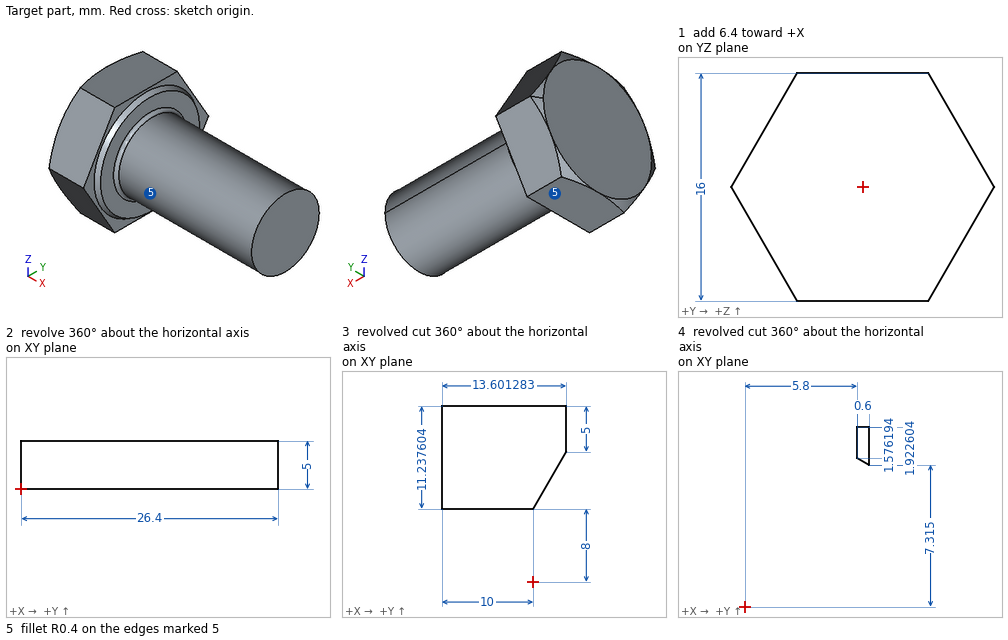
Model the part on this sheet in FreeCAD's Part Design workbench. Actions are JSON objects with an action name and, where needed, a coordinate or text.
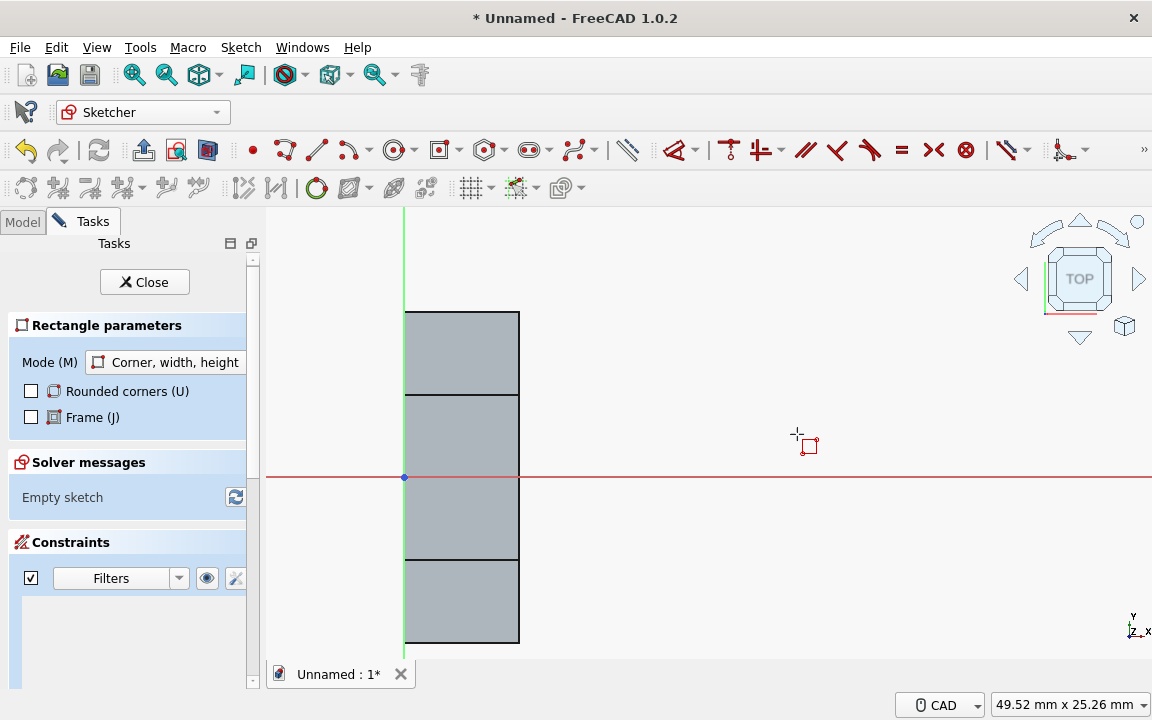
{"action": "left_click", "coordinate": [404, 477]}
{"action": "left_click", "coordinate": [876, 388]}
{"action": "key", "text": "Escape"}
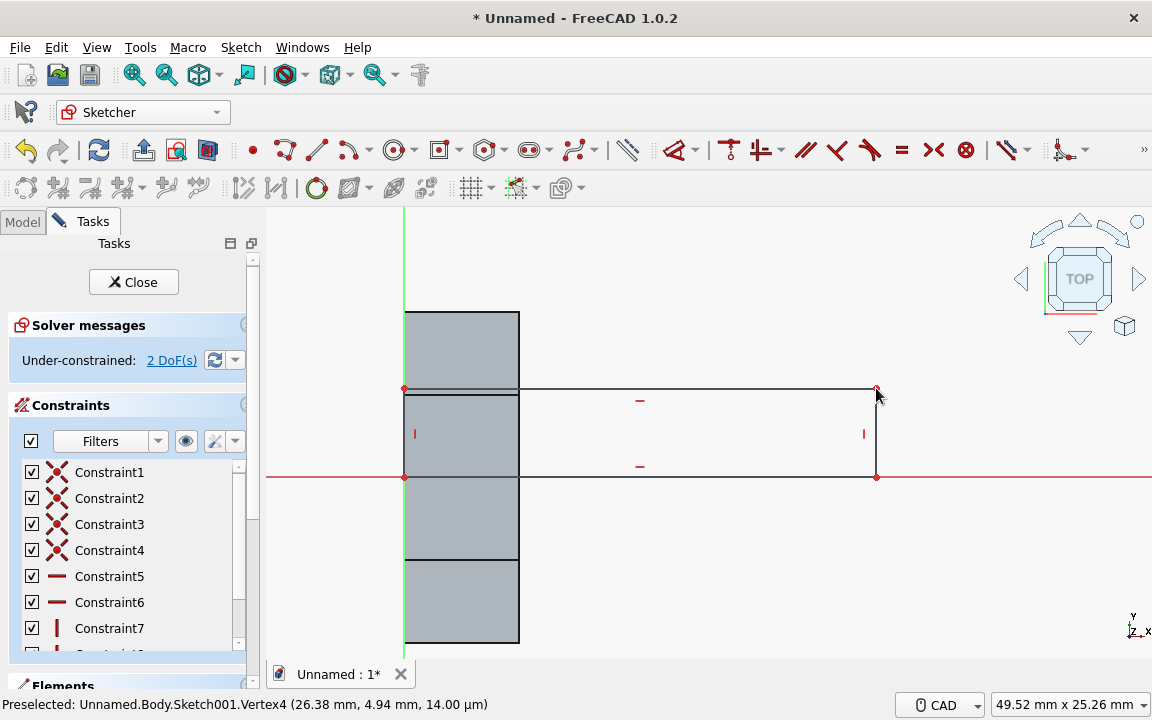
{"action": "left_click", "coordinate": [674, 150]}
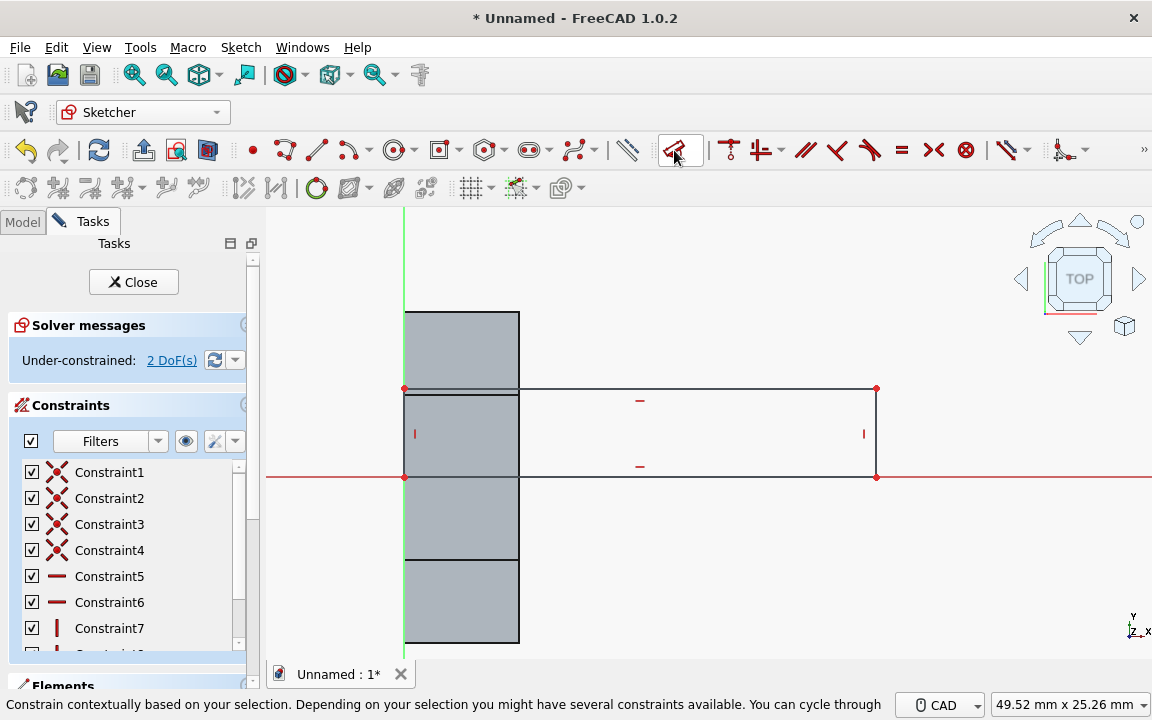
{"action": "left_click", "coordinate": [876, 451]}
{"action": "left_click", "coordinate": [910, 433]}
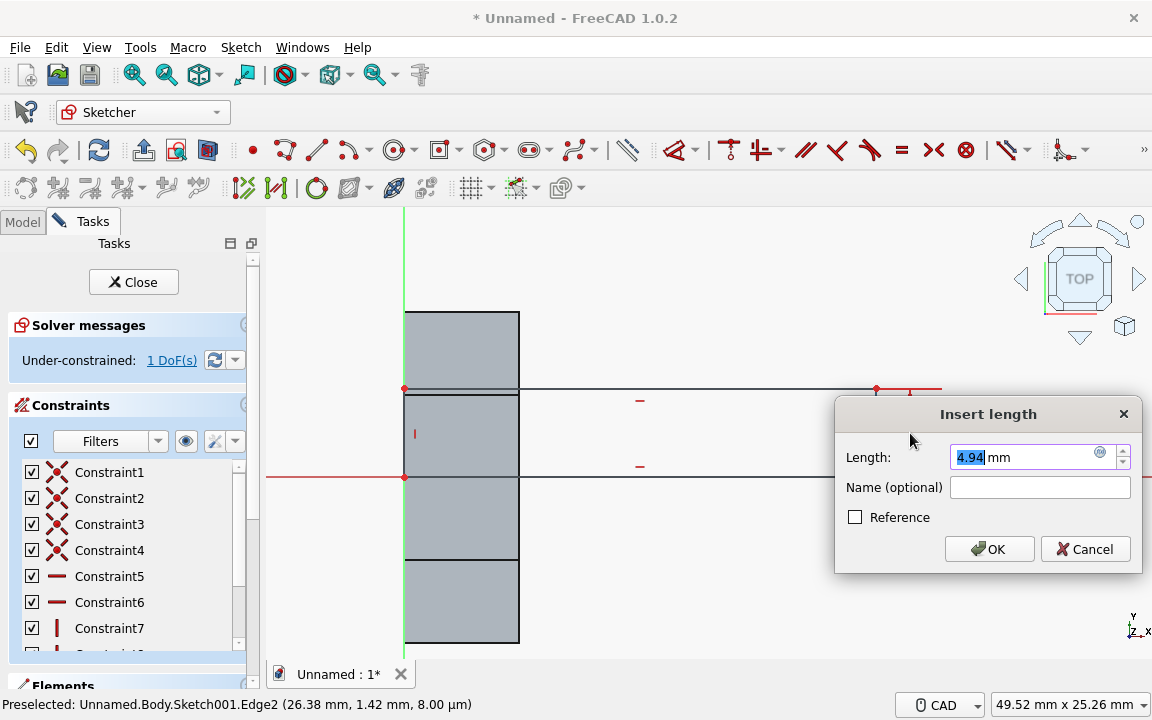
{"action": "type", "text": "5"}
{"action": "key", "text": "Return"}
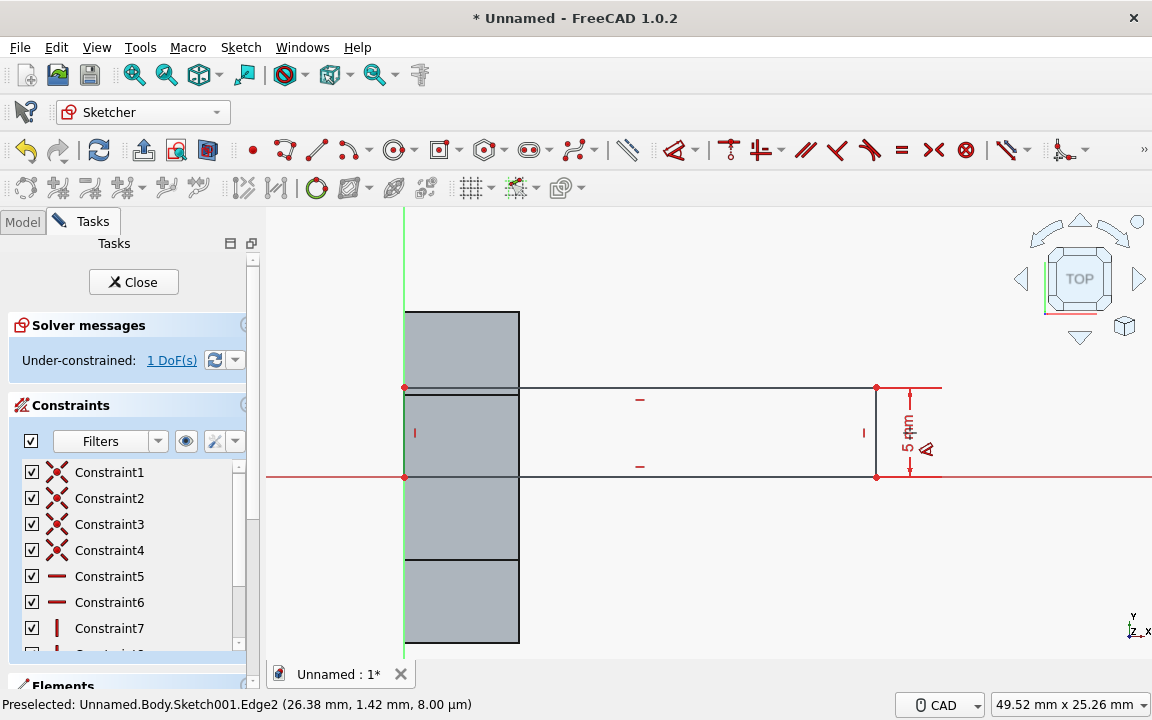
{"action": "left_click", "coordinate": [546, 477]}
{"action": "left_click", "coordinate": [640, 511]}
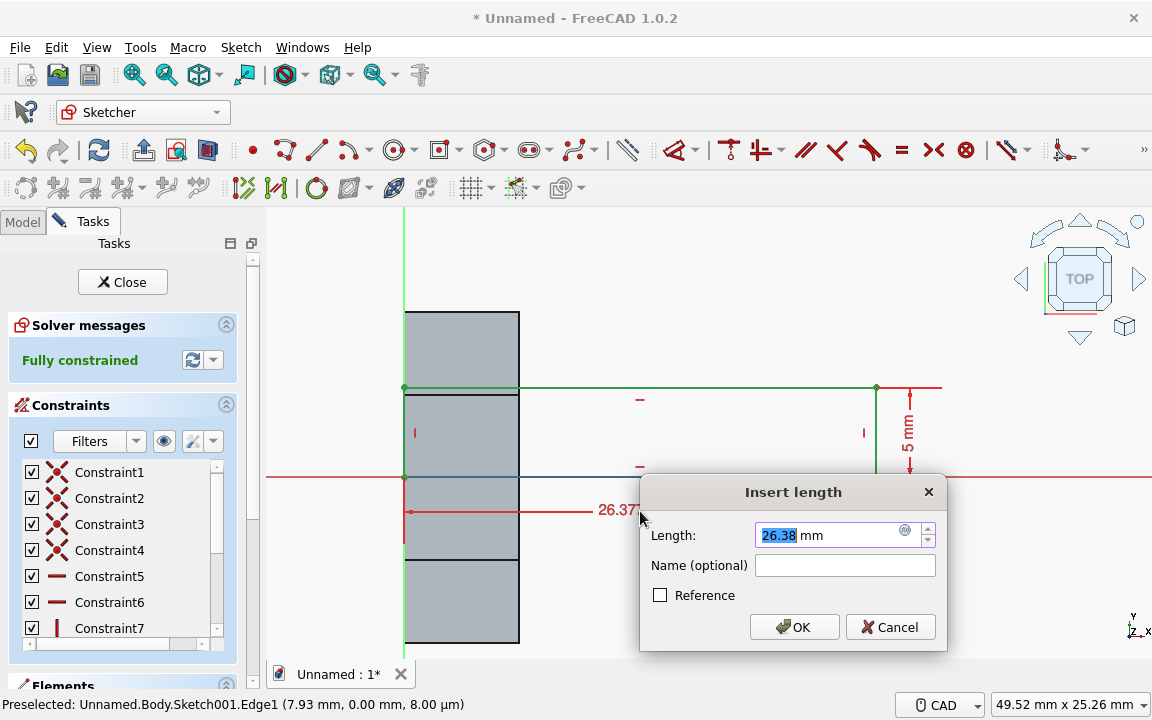
{"action": "type", "text": "26.4"}
{"action": "key", "text": "Return"}
{"action": "key", "text": "Escape"}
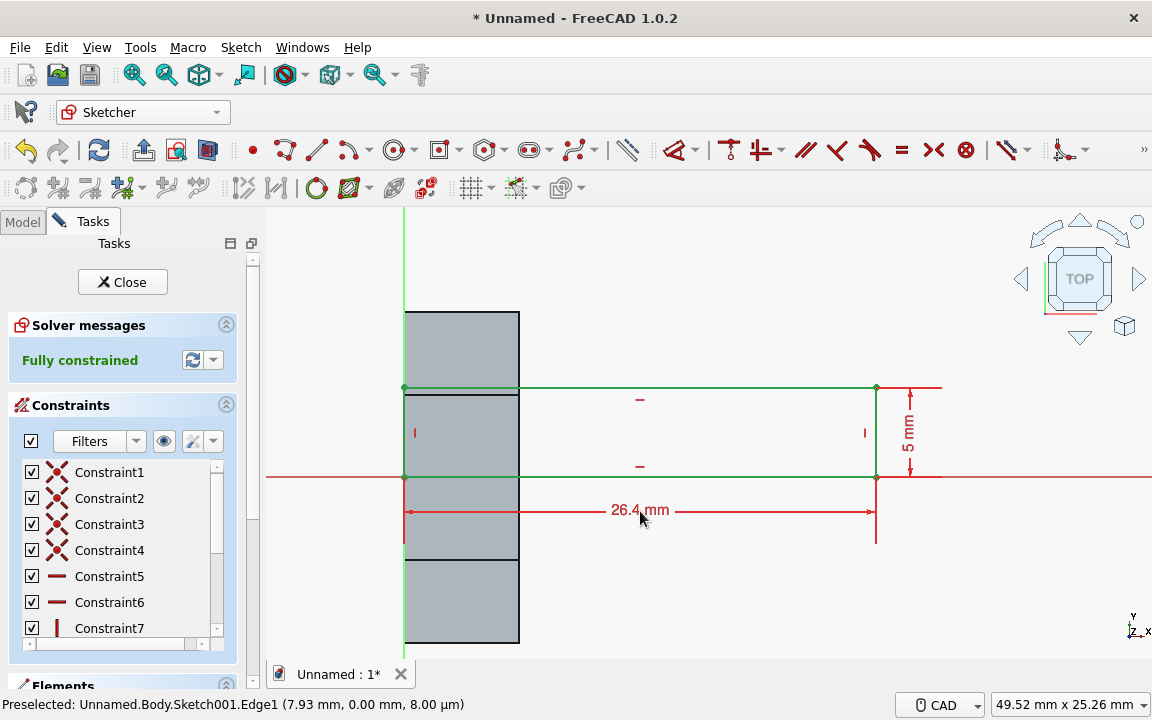
{"action": "left_click", "coordinate": [123, 282]}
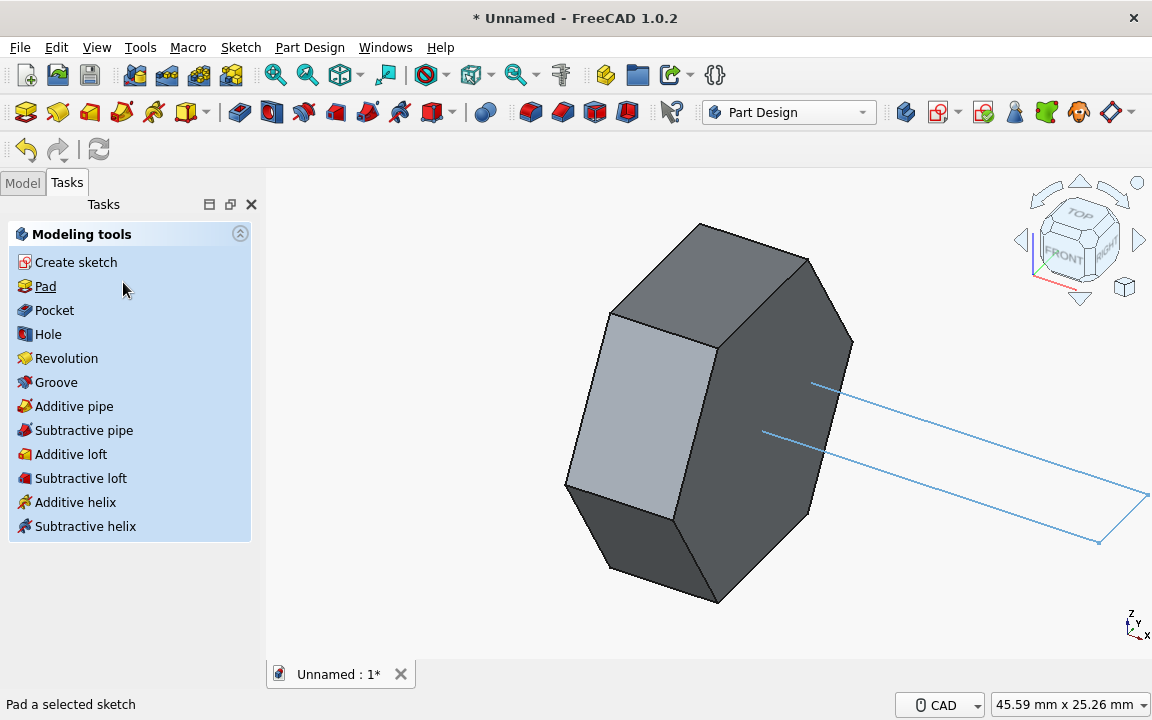
{"action": "left_click", "coordinate": [58, 112]}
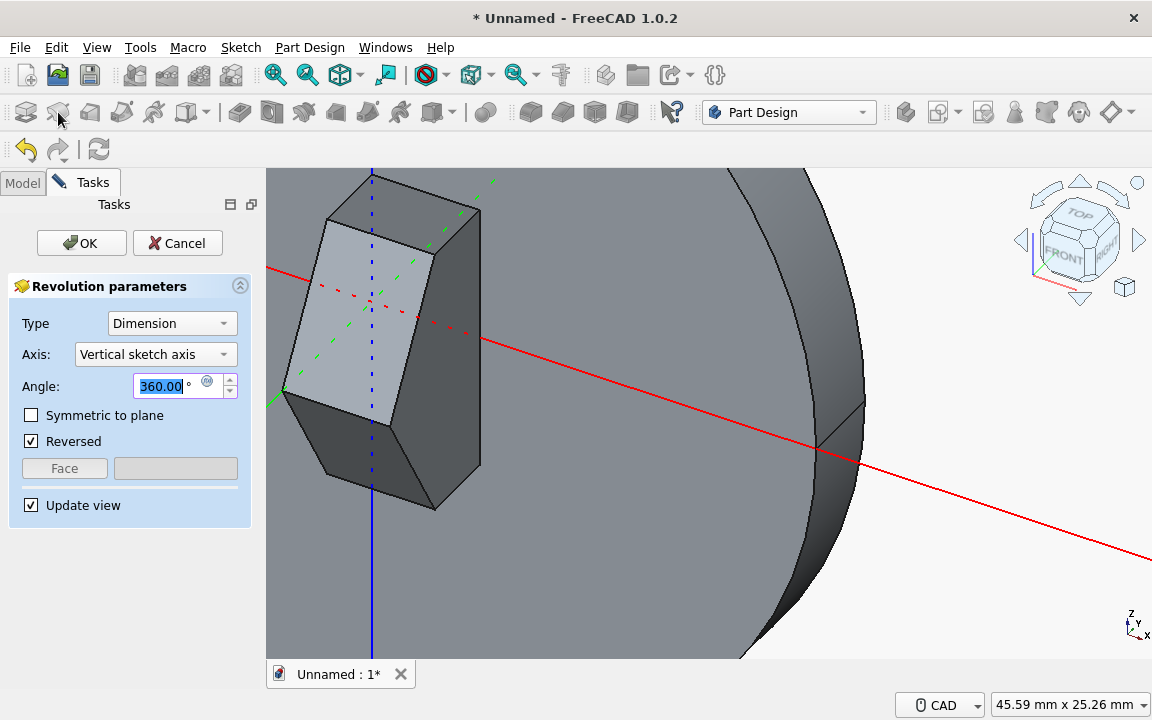
{"action": "left_click", "coordinate": [156, 354]}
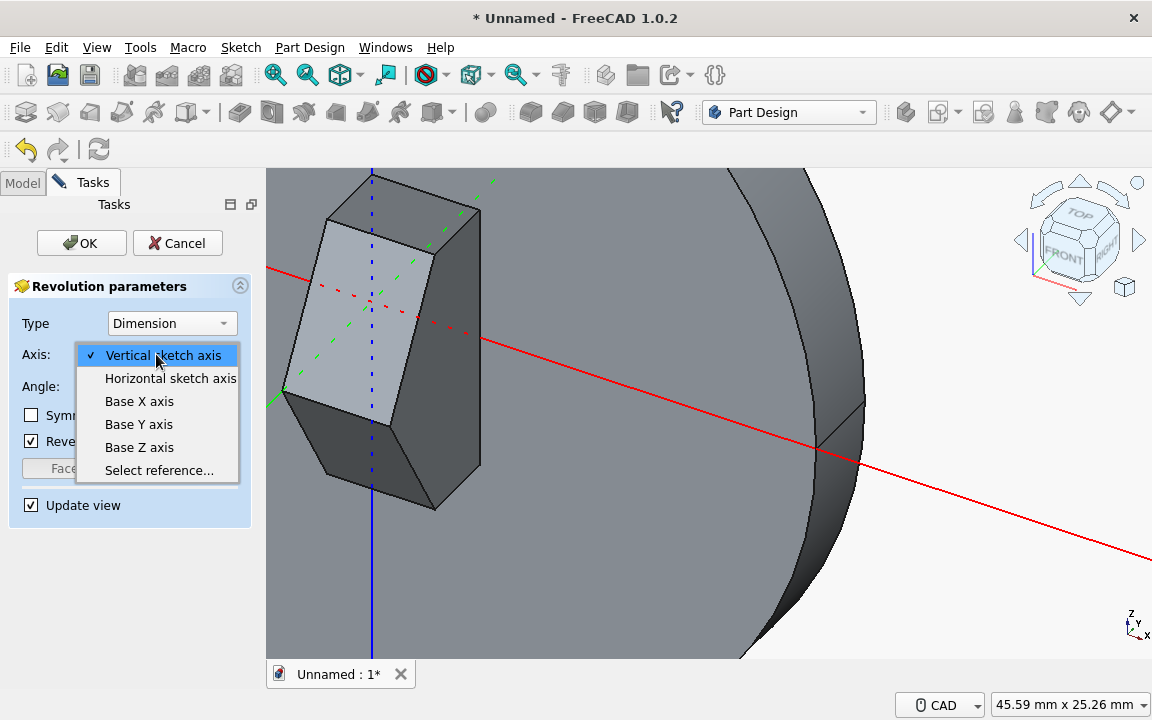
{"action": "left_click", "coordinate": [156, 378]}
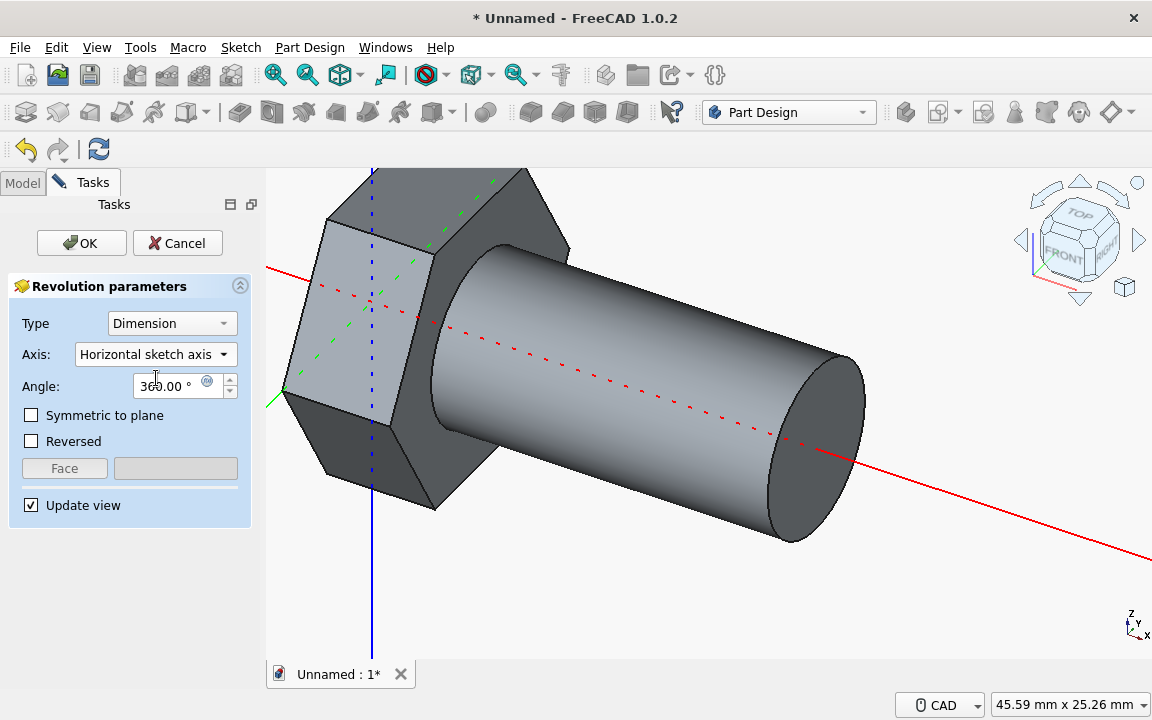
{"action": "left_click", "coordinate": [82, 243]}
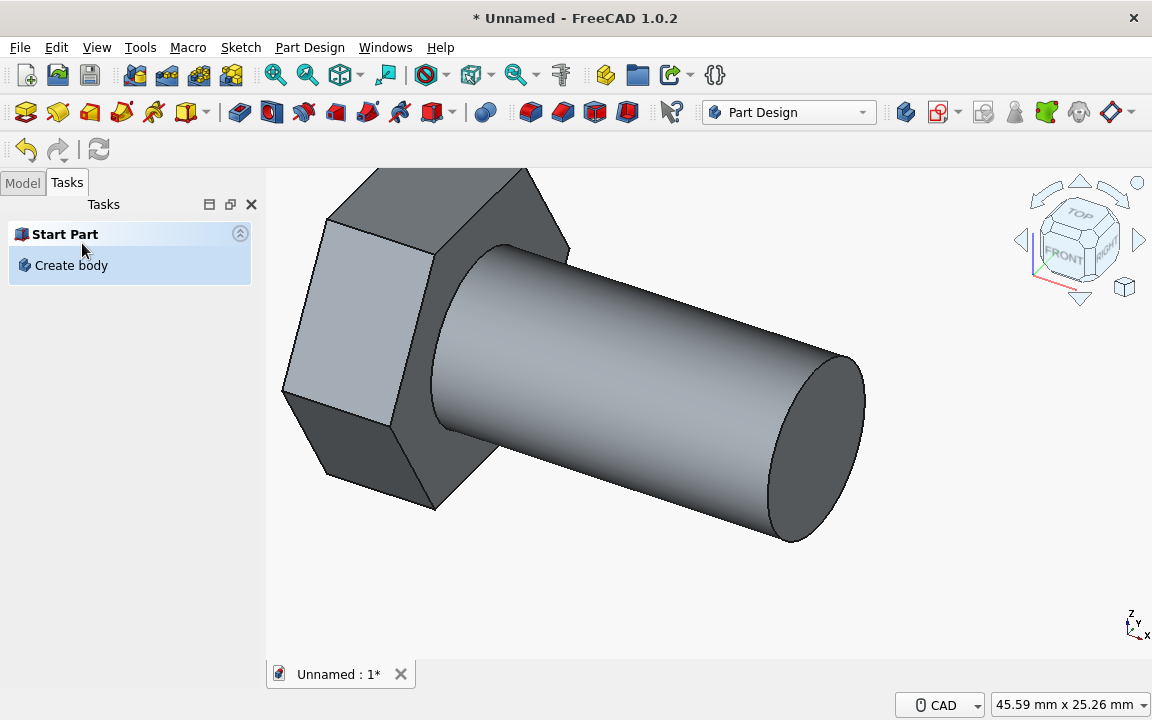
{"action": "left_click", "coordinate": [276, 76]}